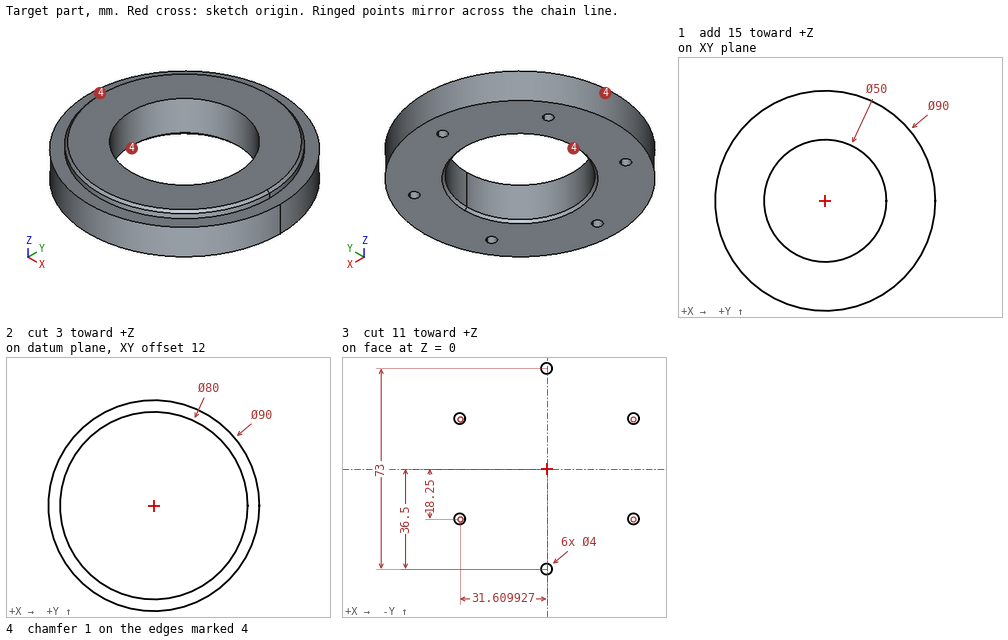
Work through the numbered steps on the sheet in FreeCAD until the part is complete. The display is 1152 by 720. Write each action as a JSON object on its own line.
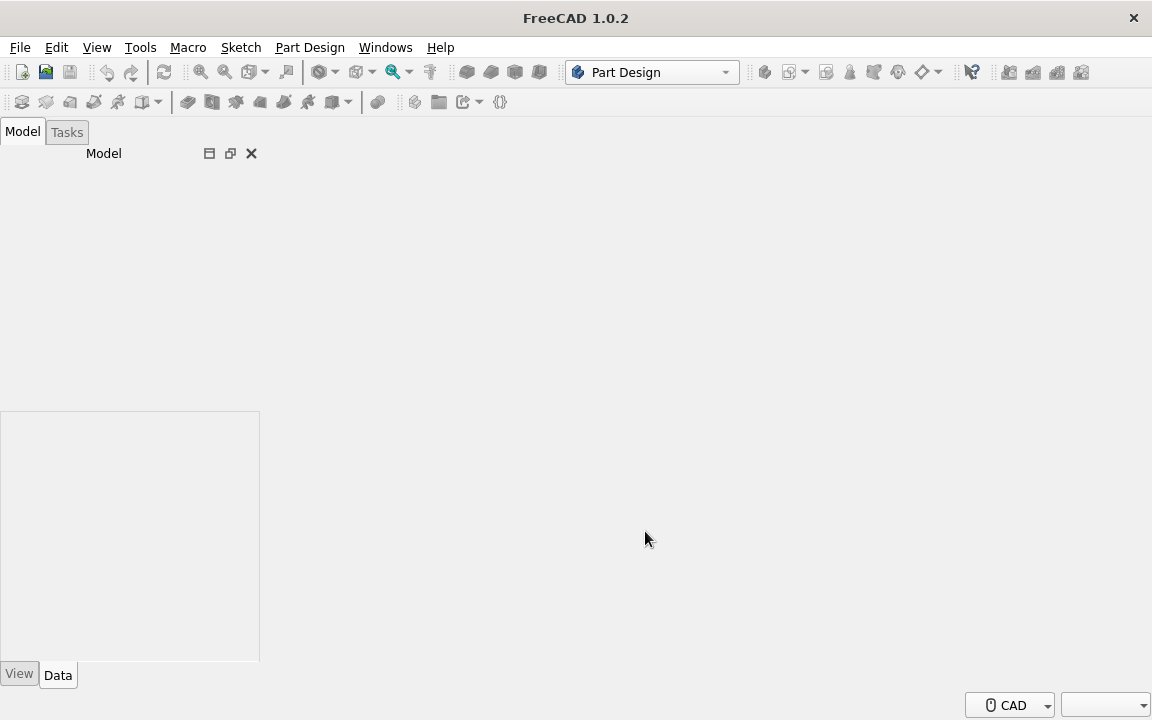
{"action": "left_click", "coordinate": [22, 72]}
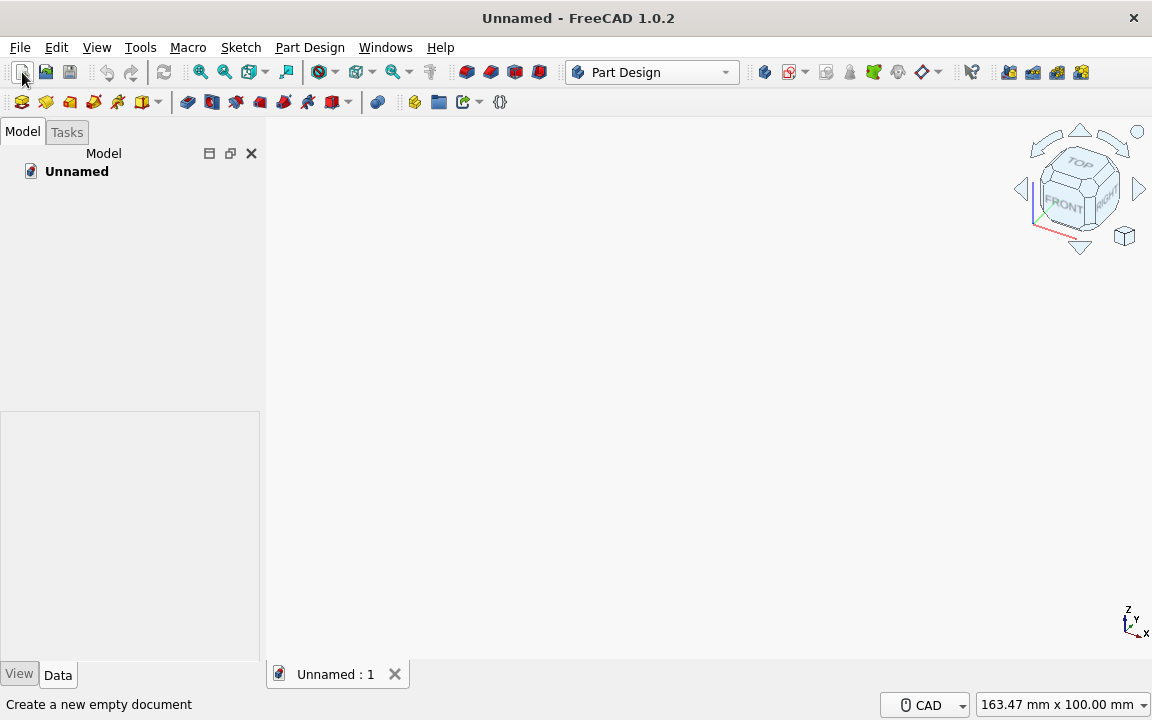
{"action": "left_click", "coordinate": [790, 72]}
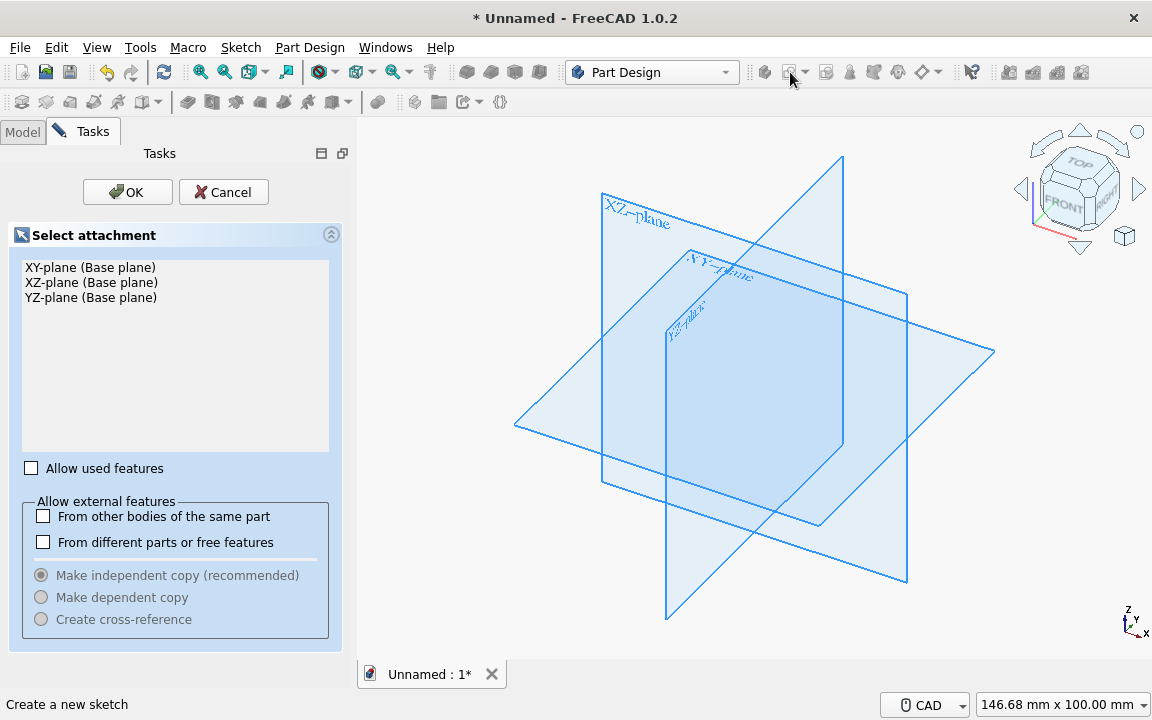
{"action": "left_click", "coordinate": [82, 268]}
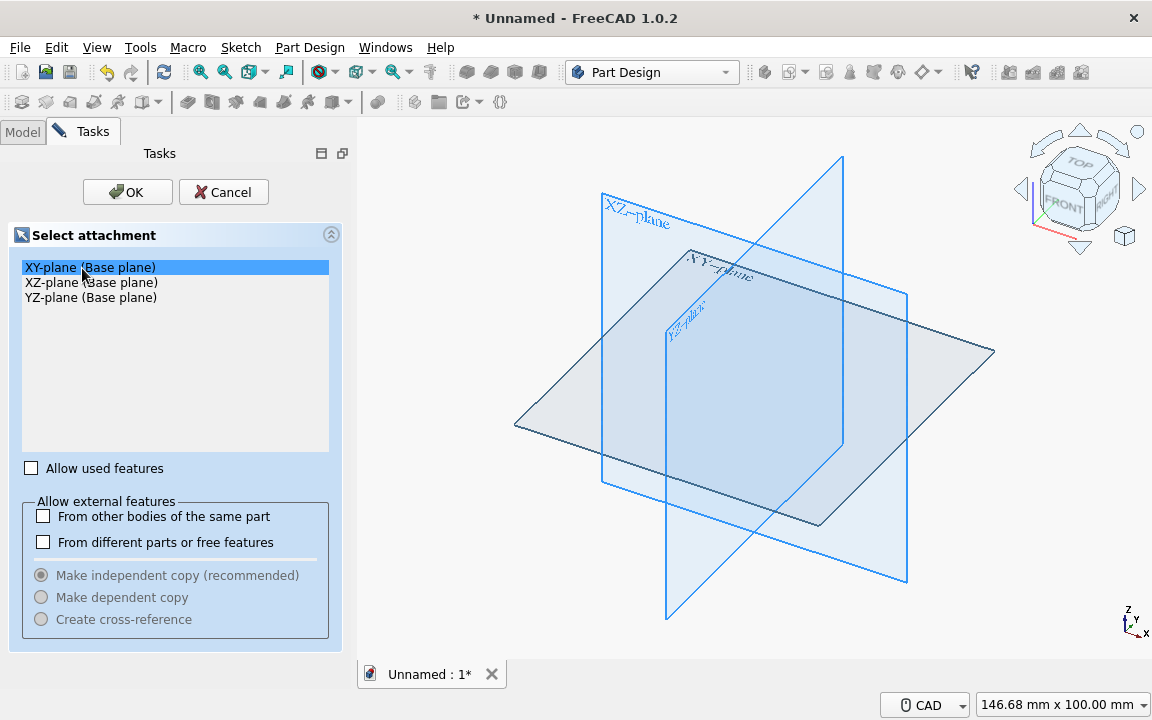
{"action": "left_click", "coordinate": [128, 192]}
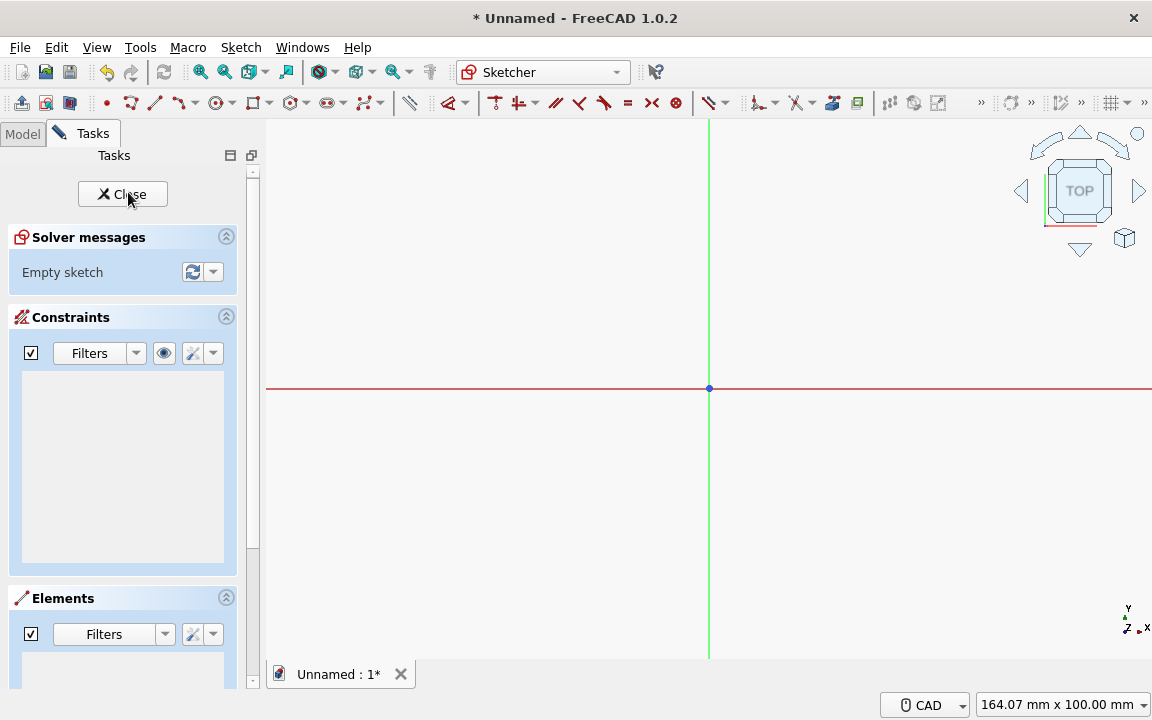
{"action": "scroll", "coordinate": [501, 389], "scroll_direction": "down", "scroll_amount": 2}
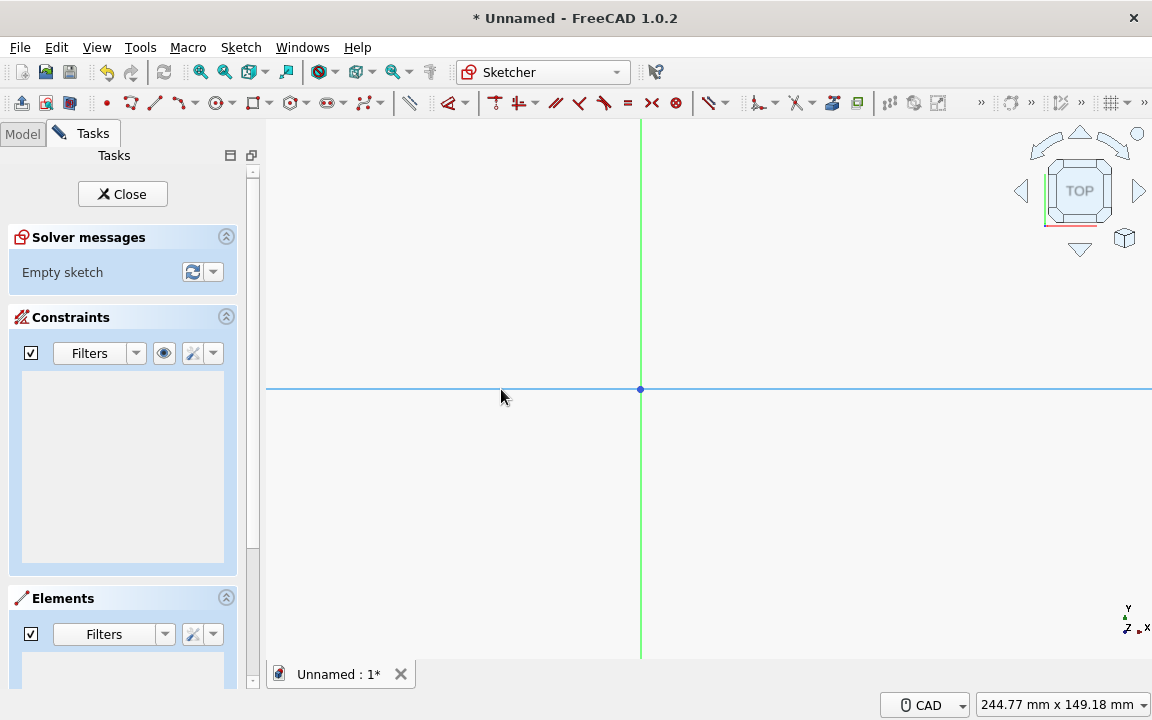
{"action": "left_click", "coordinate": [216, 104]}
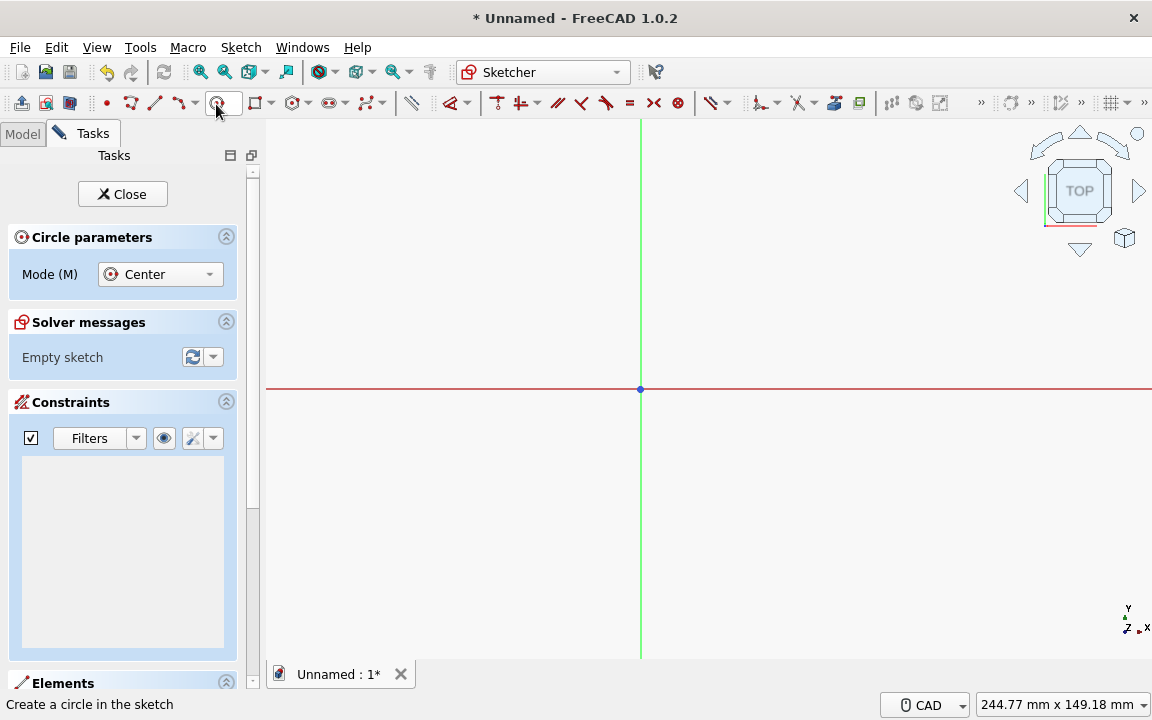
{"action": "left_click", "coordinate": [641, 389]}
{"action": "left_click", "coordinate": [756, 274]}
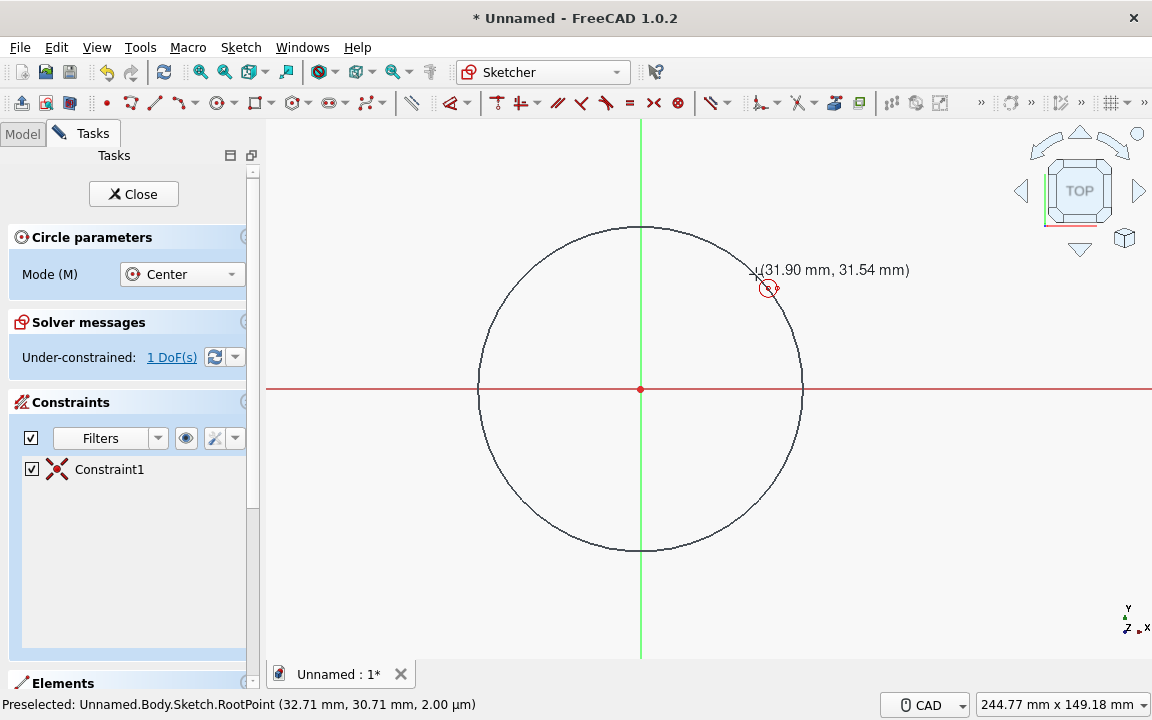
{"action": "left_click", "coordinate": [641, 389]}
{"action": "left_click", "coordinate": [705, 325]}
{"action": "key", "text": "Escape"}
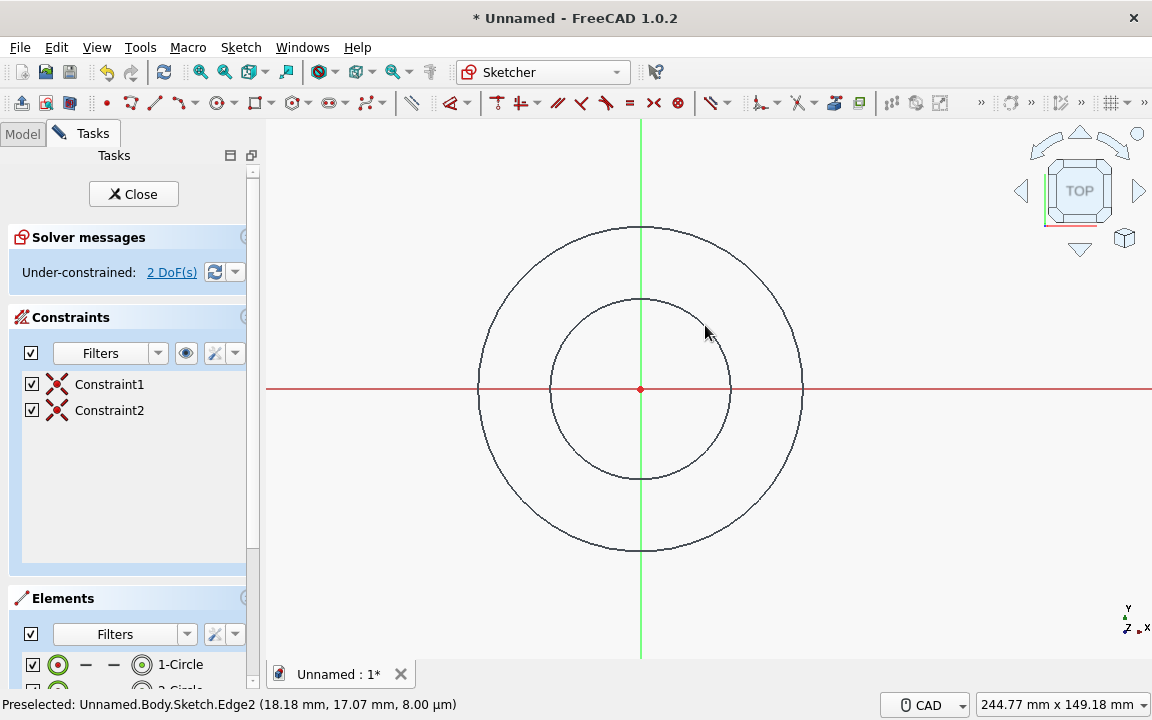
{"action": "key", "text": "d"}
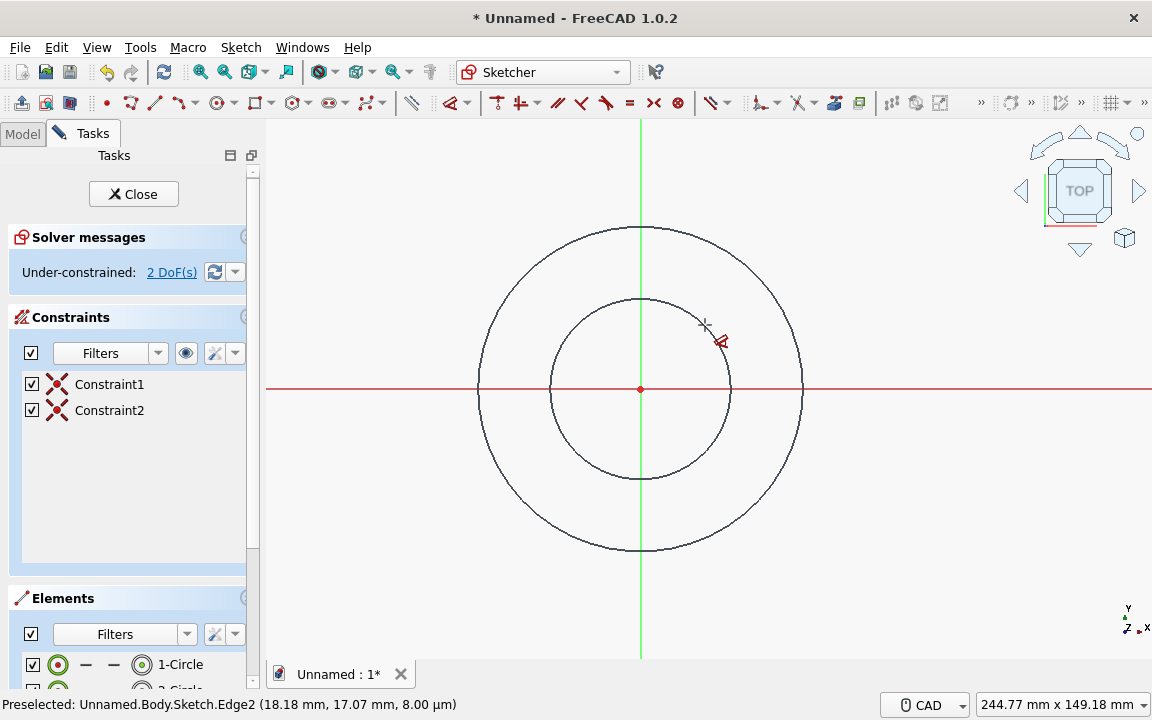
{"action": "left_click", "coordinate": [755, 274]}
{"action": "left_click", "coordinate": [778, 251]}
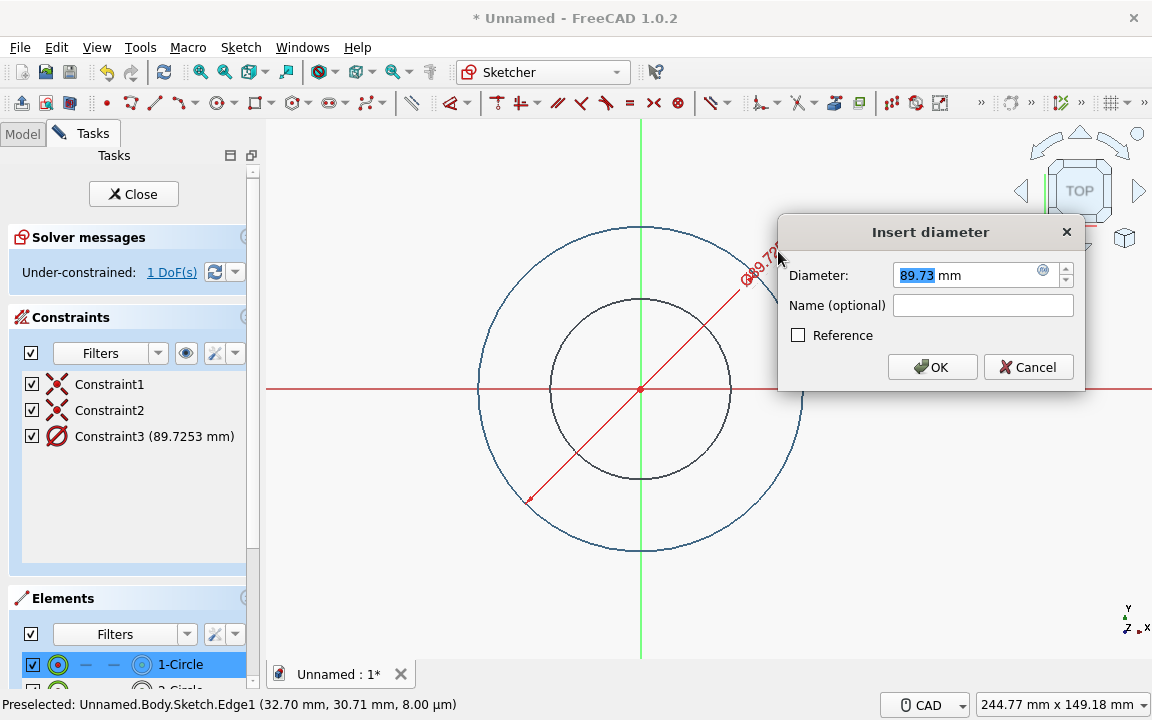
{"action": "type", "text": "90"}
{"action": "key", "text": "Return"}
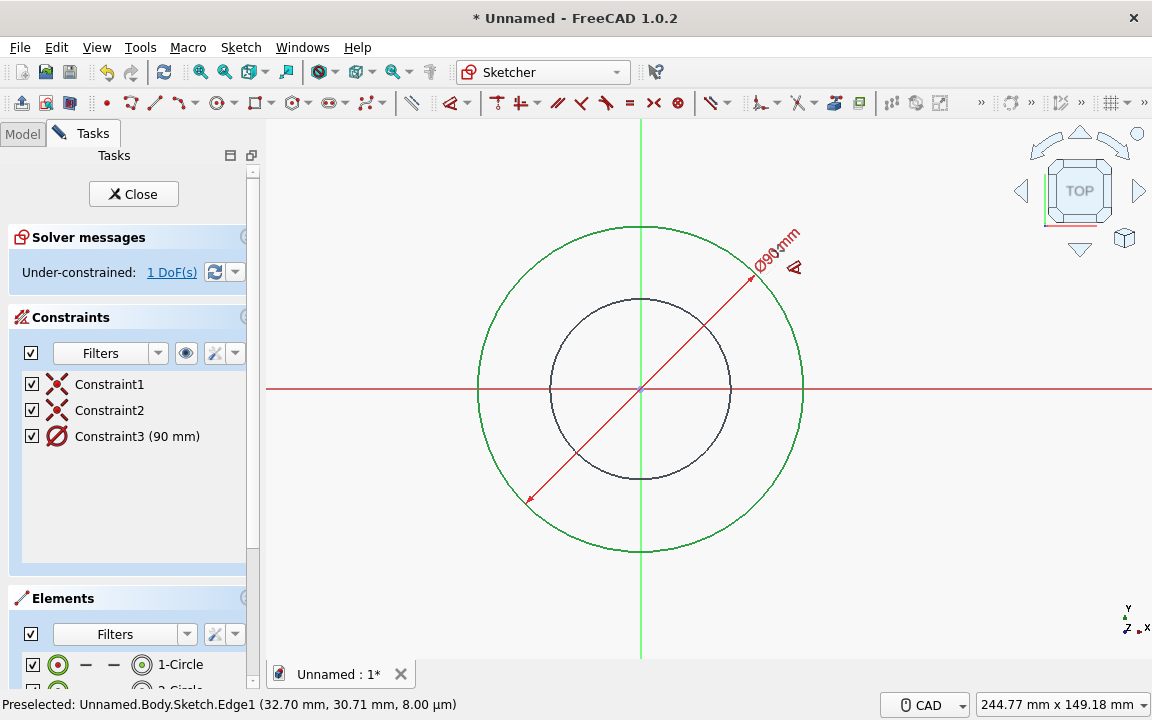
{"action": "left_click", "coordinate": [704, 325]}
{"action": "left_click", "coordinate": [727, 302]}